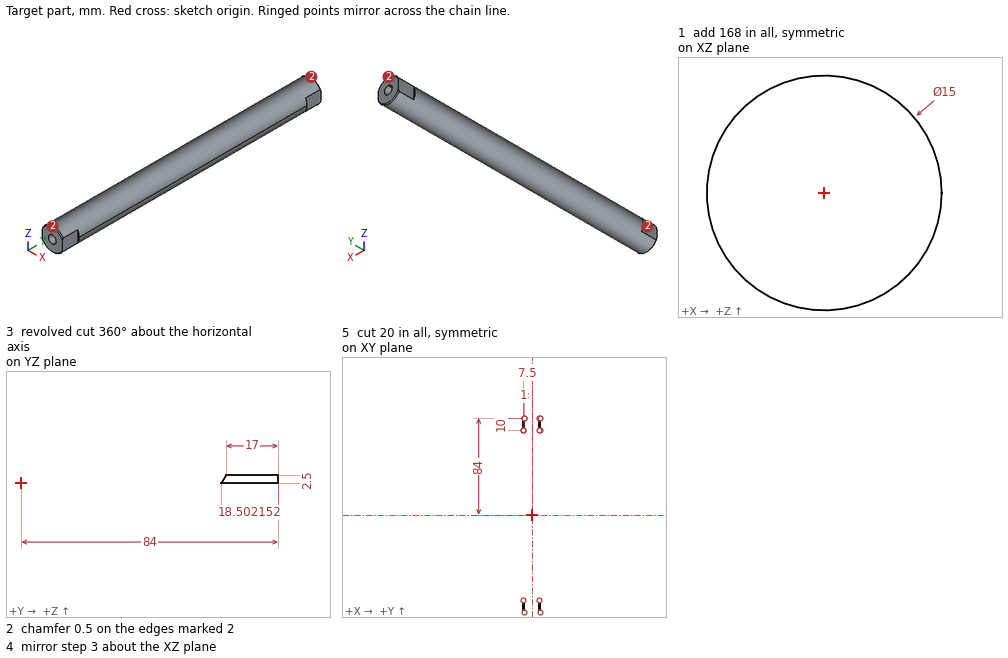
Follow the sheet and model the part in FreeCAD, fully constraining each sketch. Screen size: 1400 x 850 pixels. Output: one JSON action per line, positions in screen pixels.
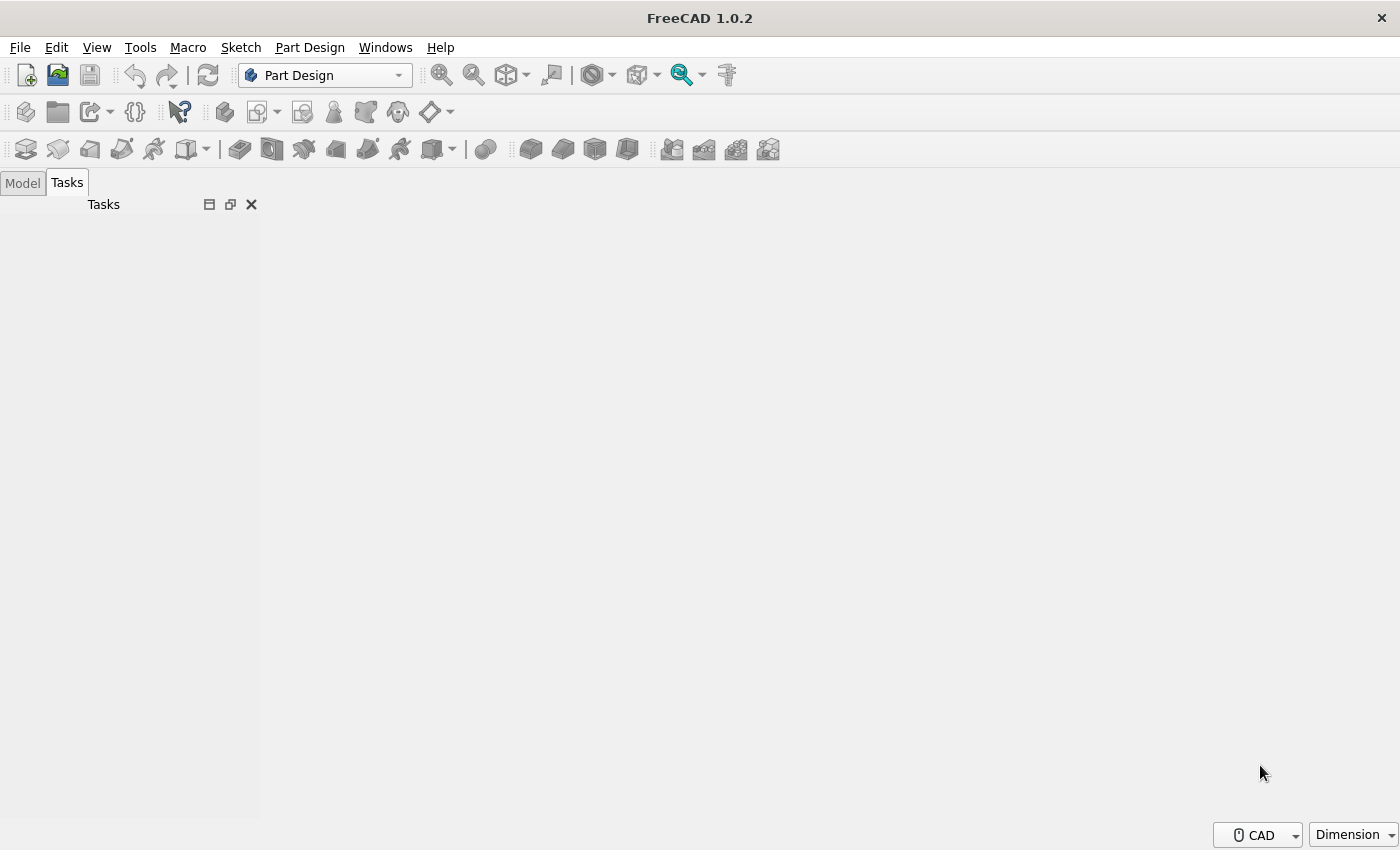
{"action": "left_click", "coordinate": [26, 76]}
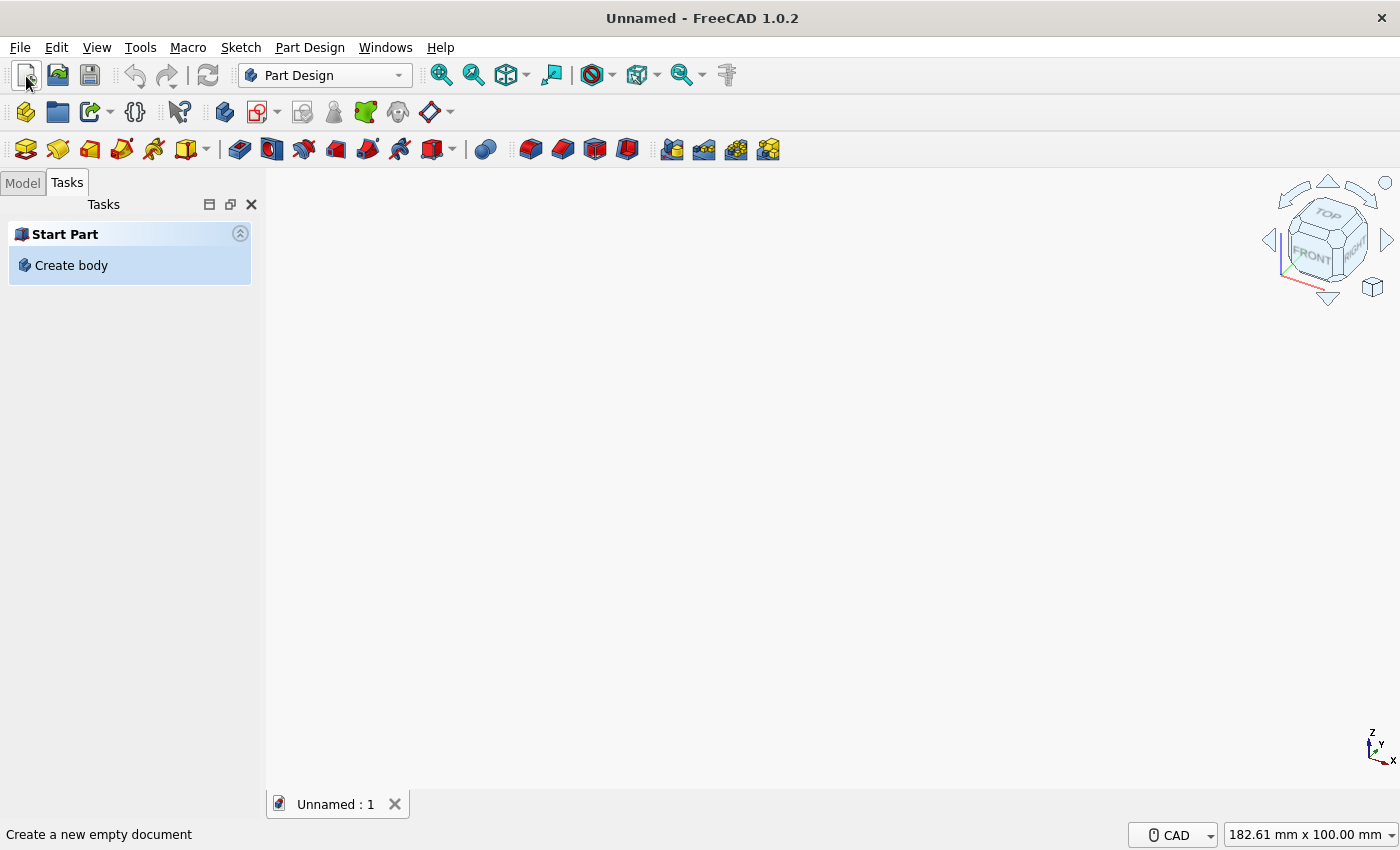
{"action": "left_click", "coordinate": [258, 112]}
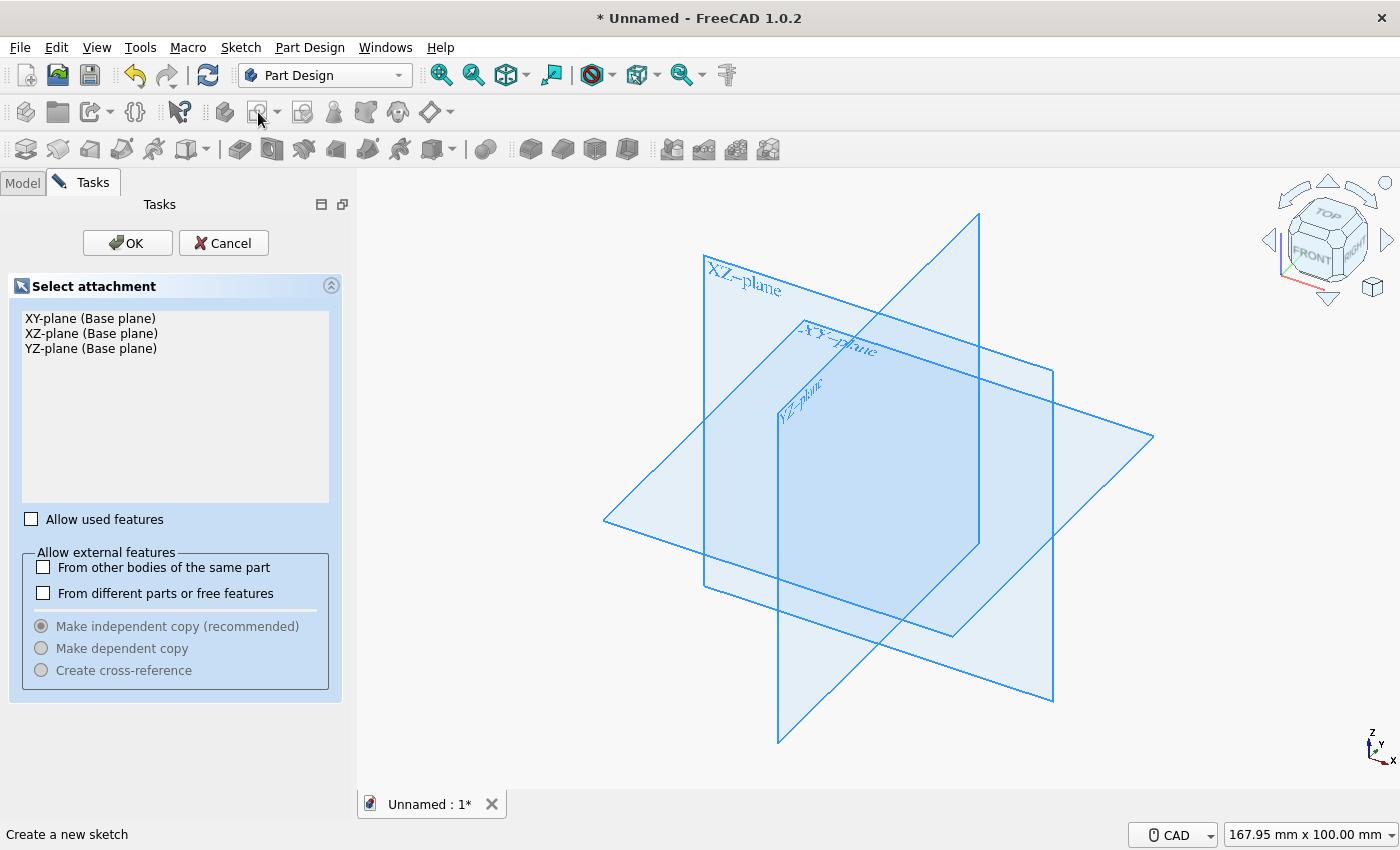
{"action": "left_click", "coordinate": [82, 334]}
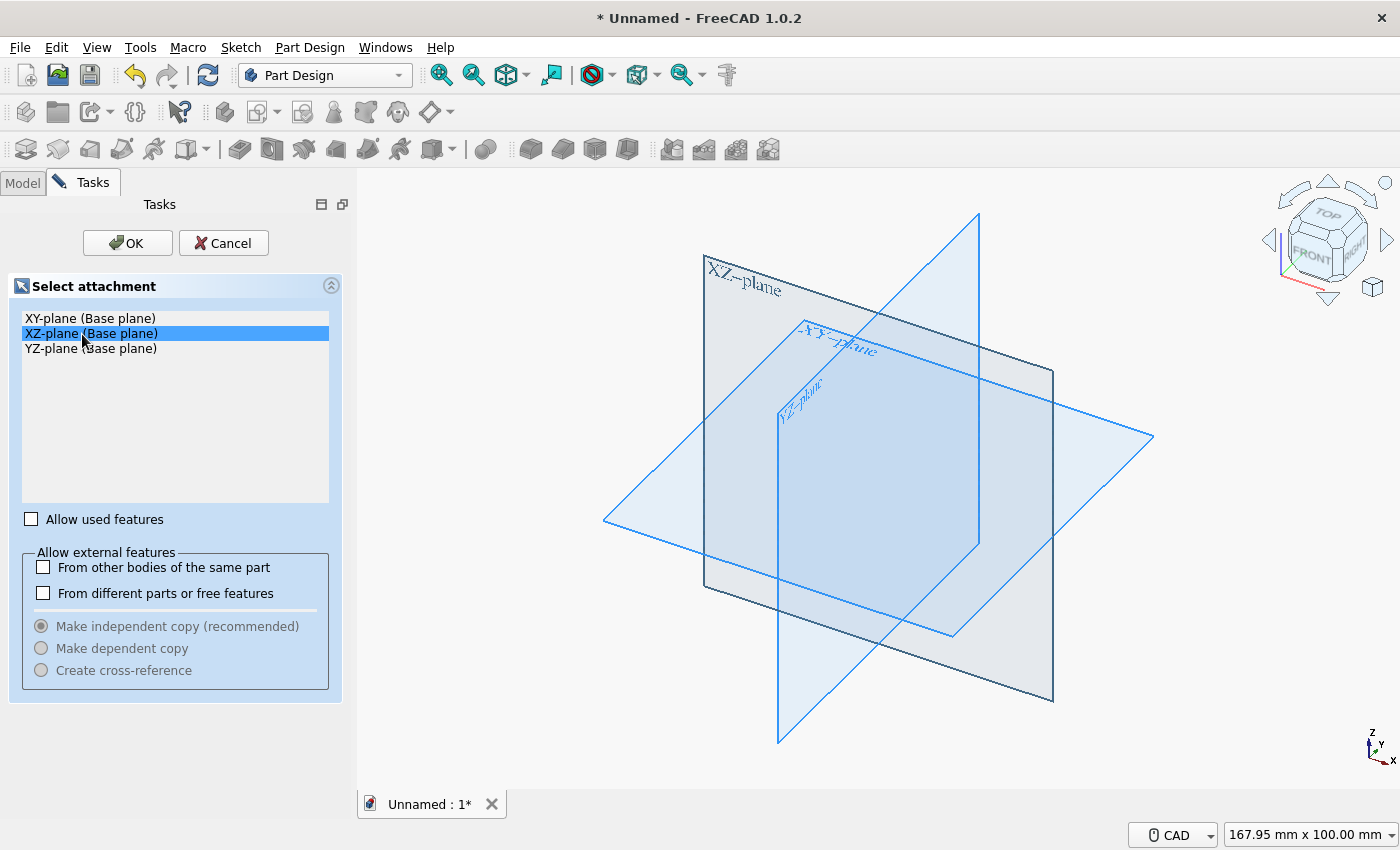
{"action": "left_click", "coordinate": [128, 243]}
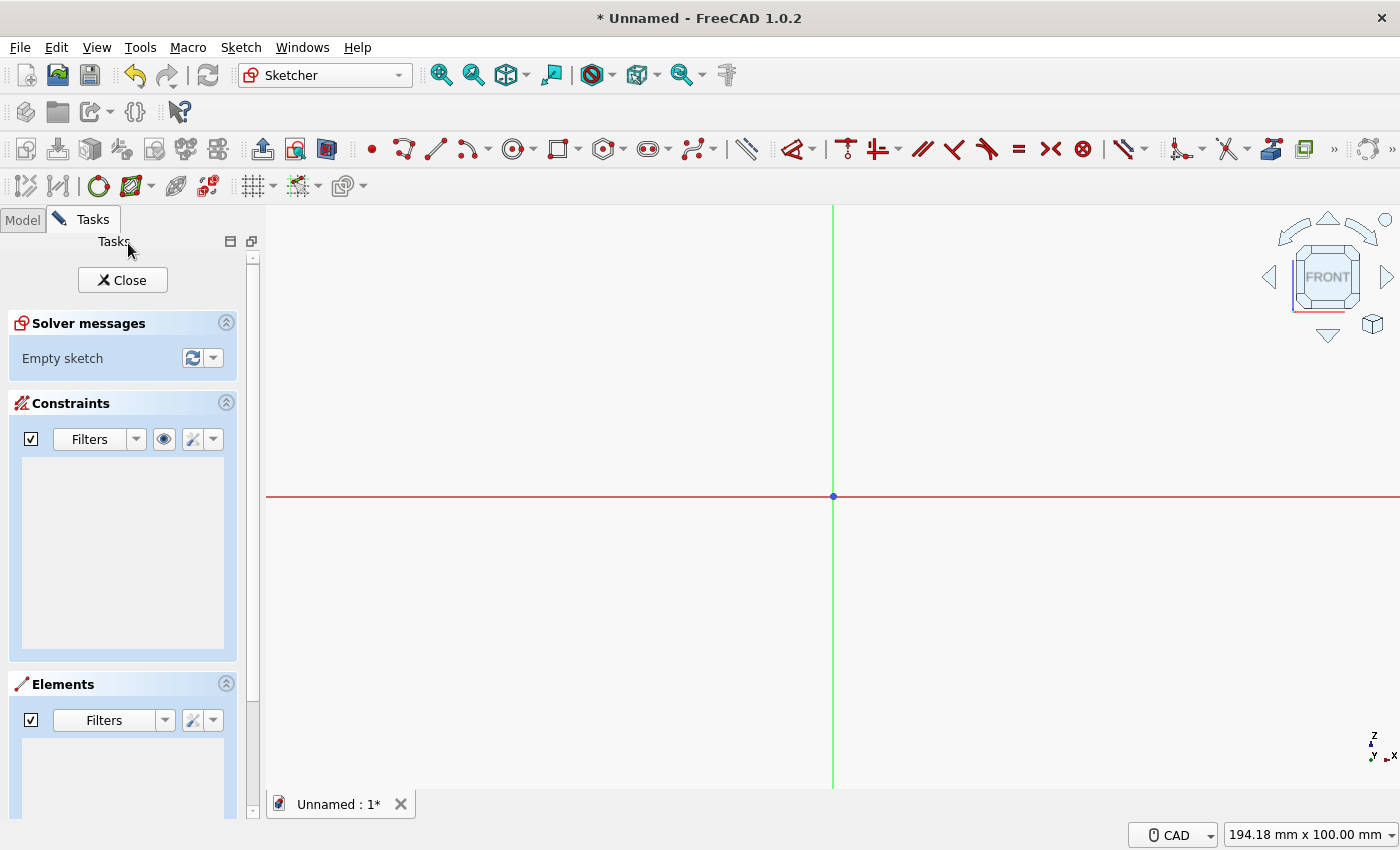
{"action": "scroll", "coordinate": [855, 497], "scroll_direction": "up", "scroll_amount": 7}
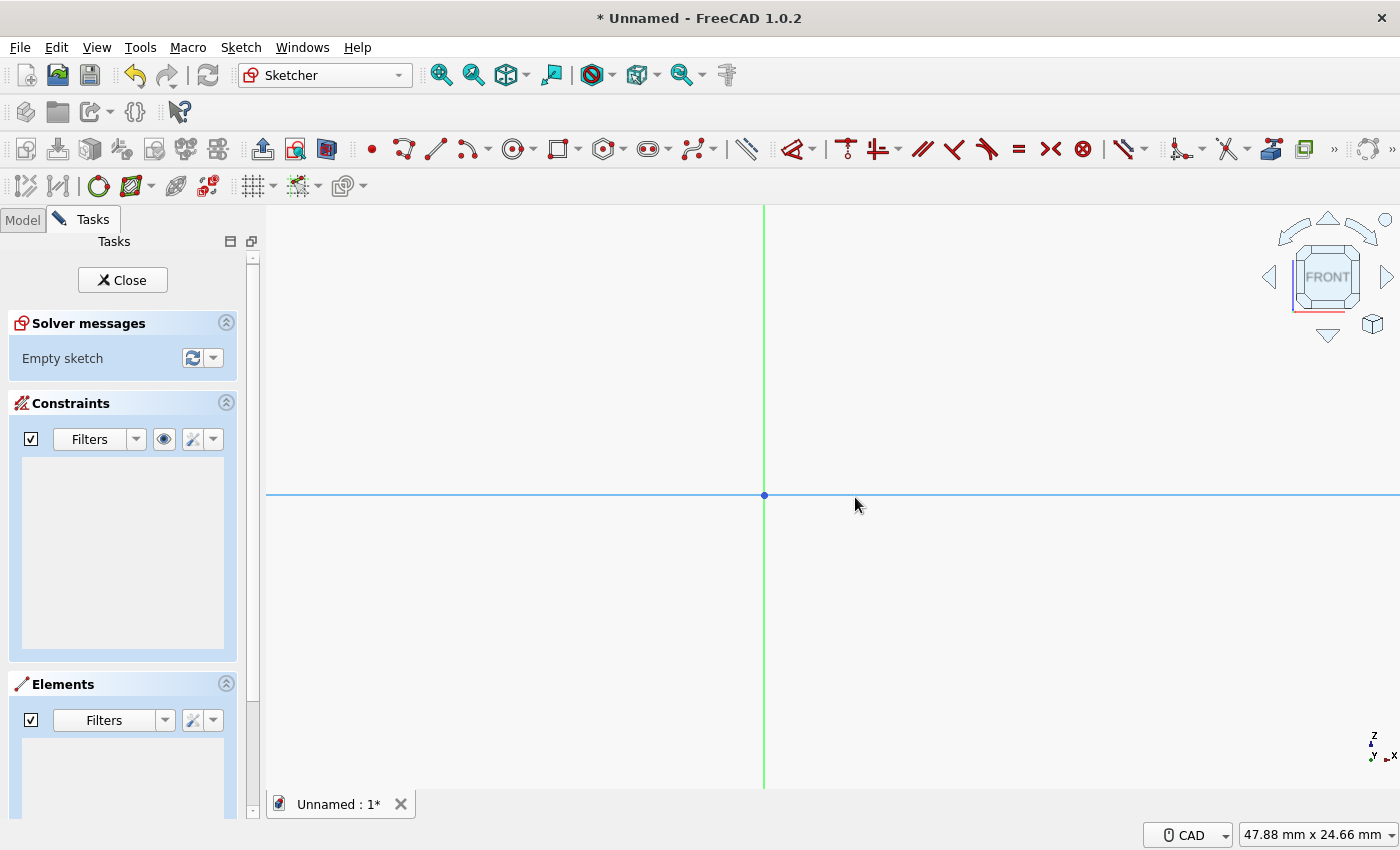
{"action": "left_click", "coordinate": [514, 150]}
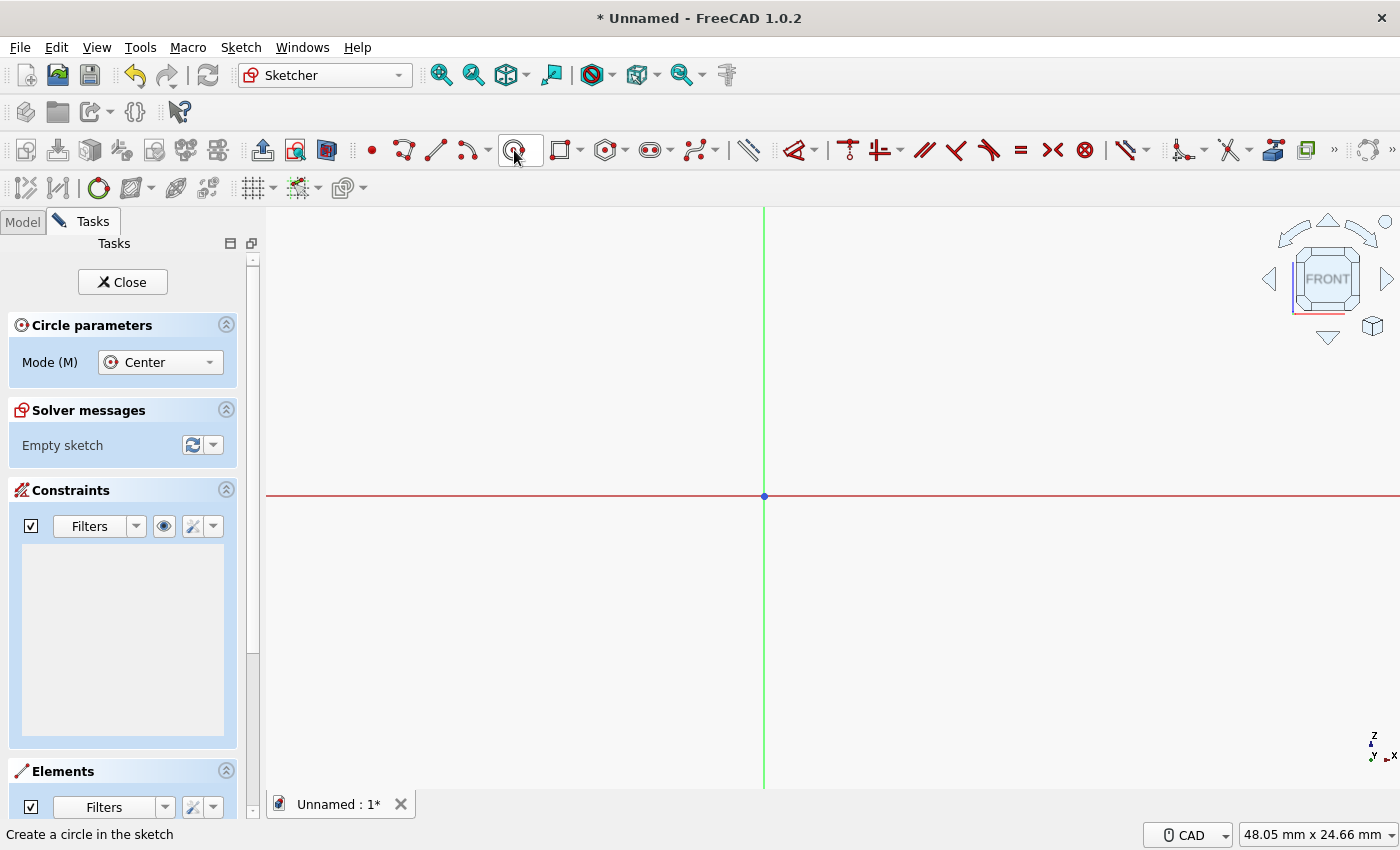
{"action": "left_click", "coordinate": [764, 496]}
{"action": "left_click", "coordinate": [890, 371]}
{"action": "key", "text": "Escape"}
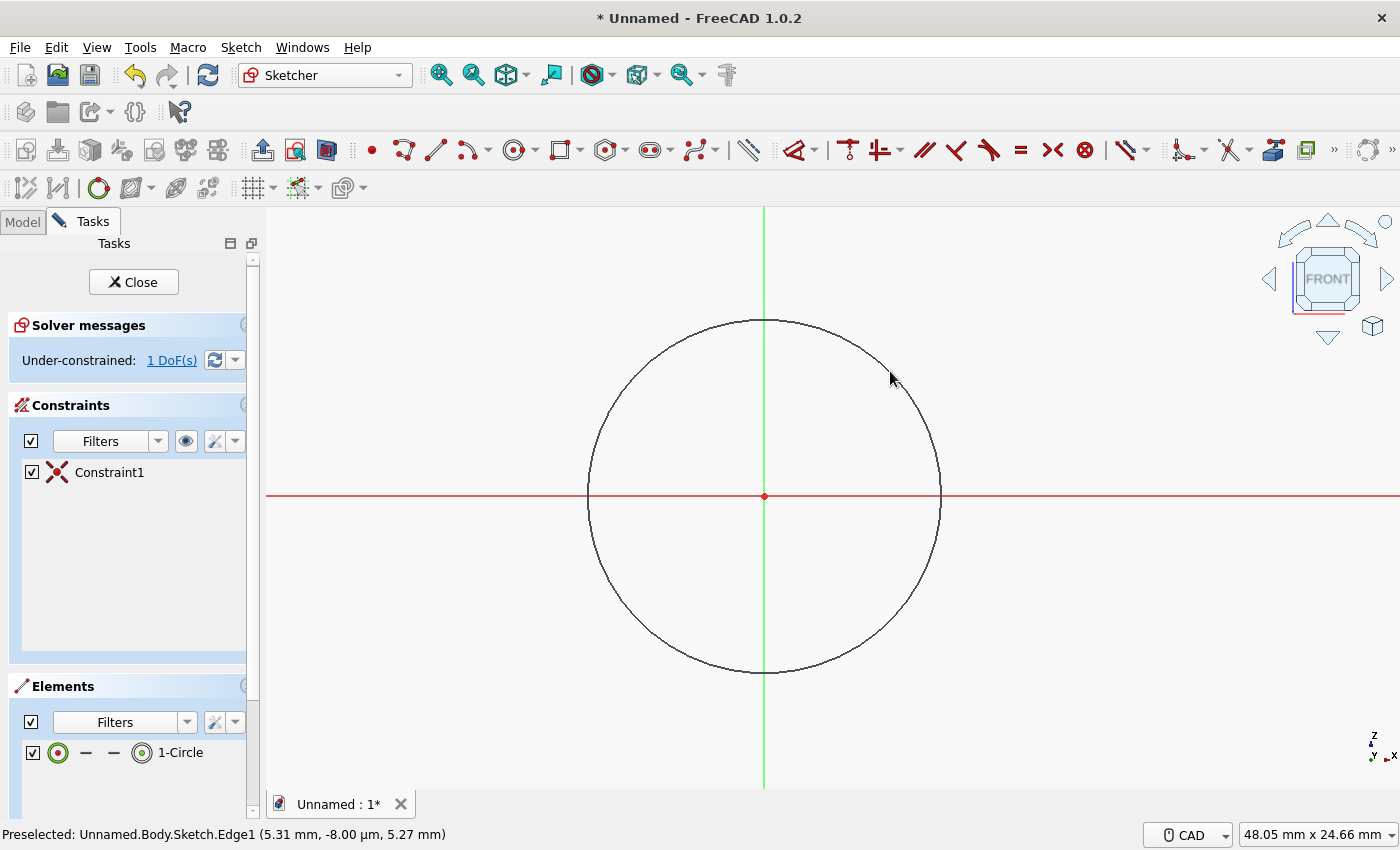
{"action": "left_click", "coordinate": [794, 150]}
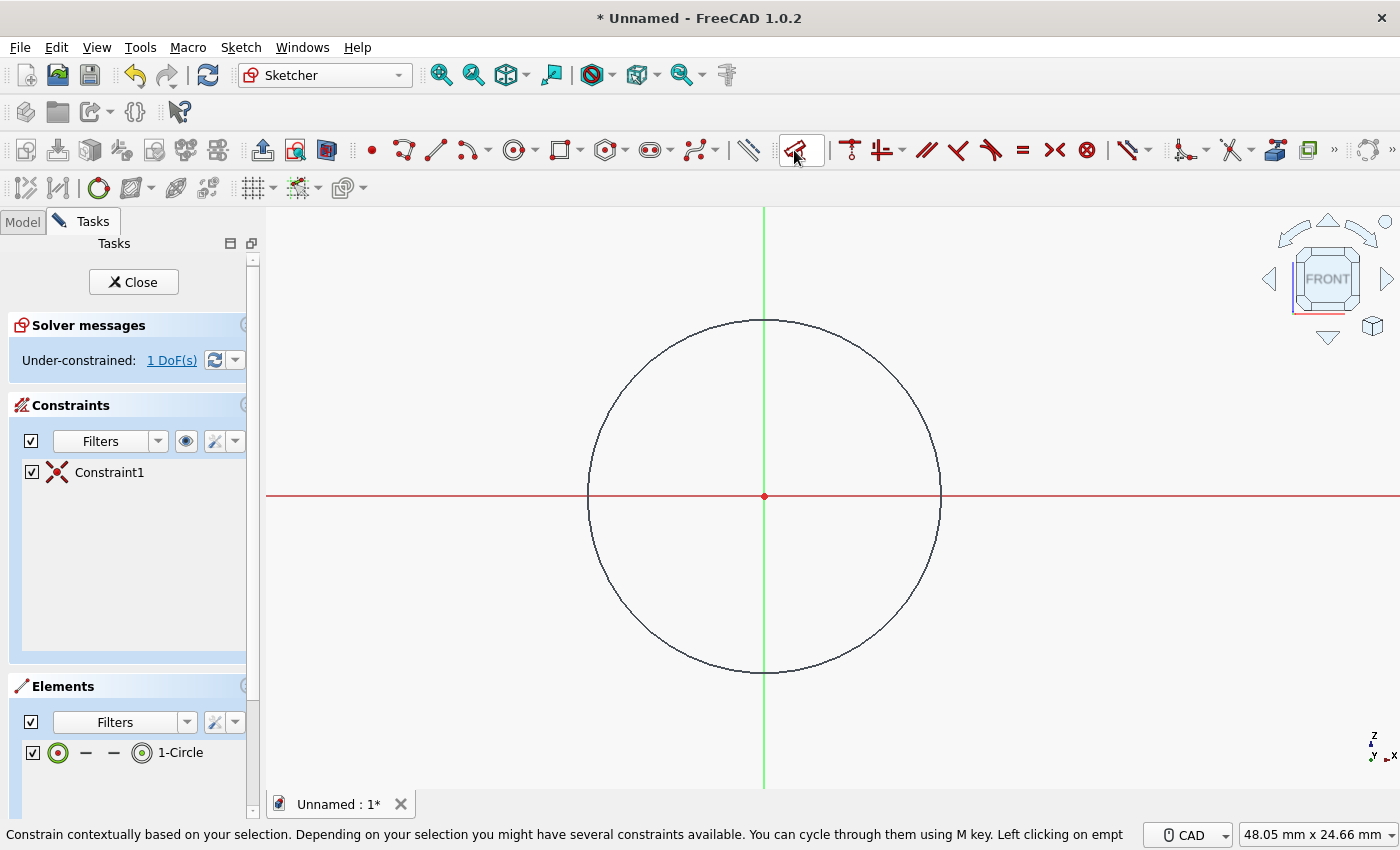
{"action": "left_click", "coordinate": [889, 371]}
{"action": "left_click", "coordinate": [912, 348]}